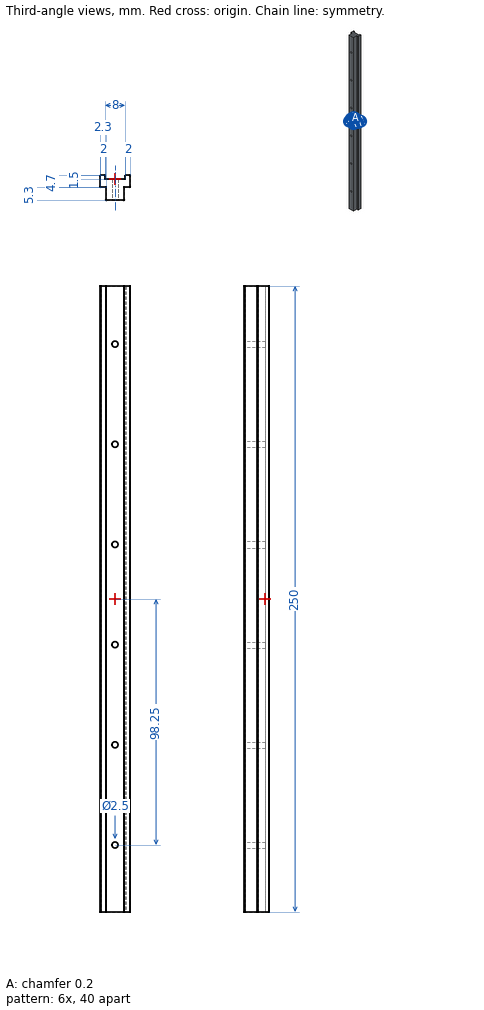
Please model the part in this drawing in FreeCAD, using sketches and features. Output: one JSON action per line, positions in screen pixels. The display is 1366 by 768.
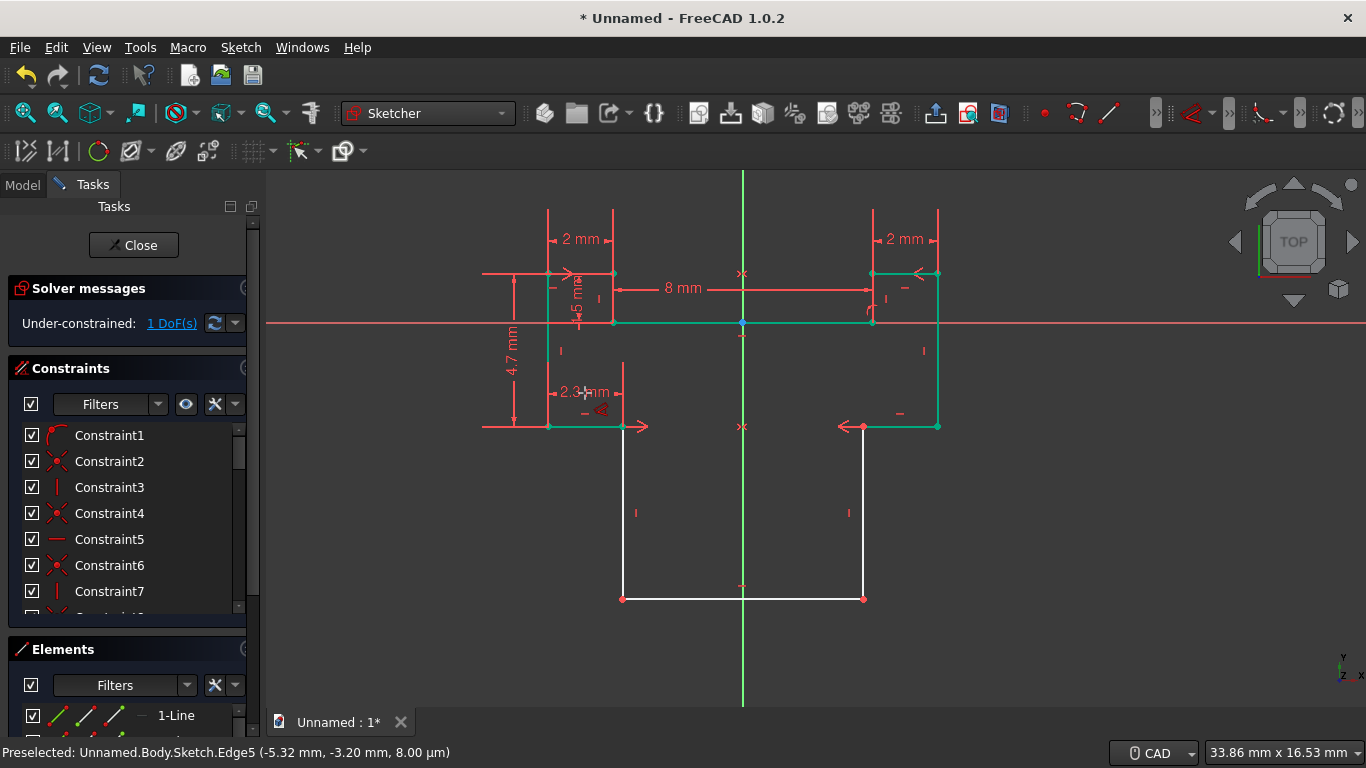
{"action": "left_click", "coordinate": [623, 478]}
{"action": "left_click", "coordinate": [589, 513]}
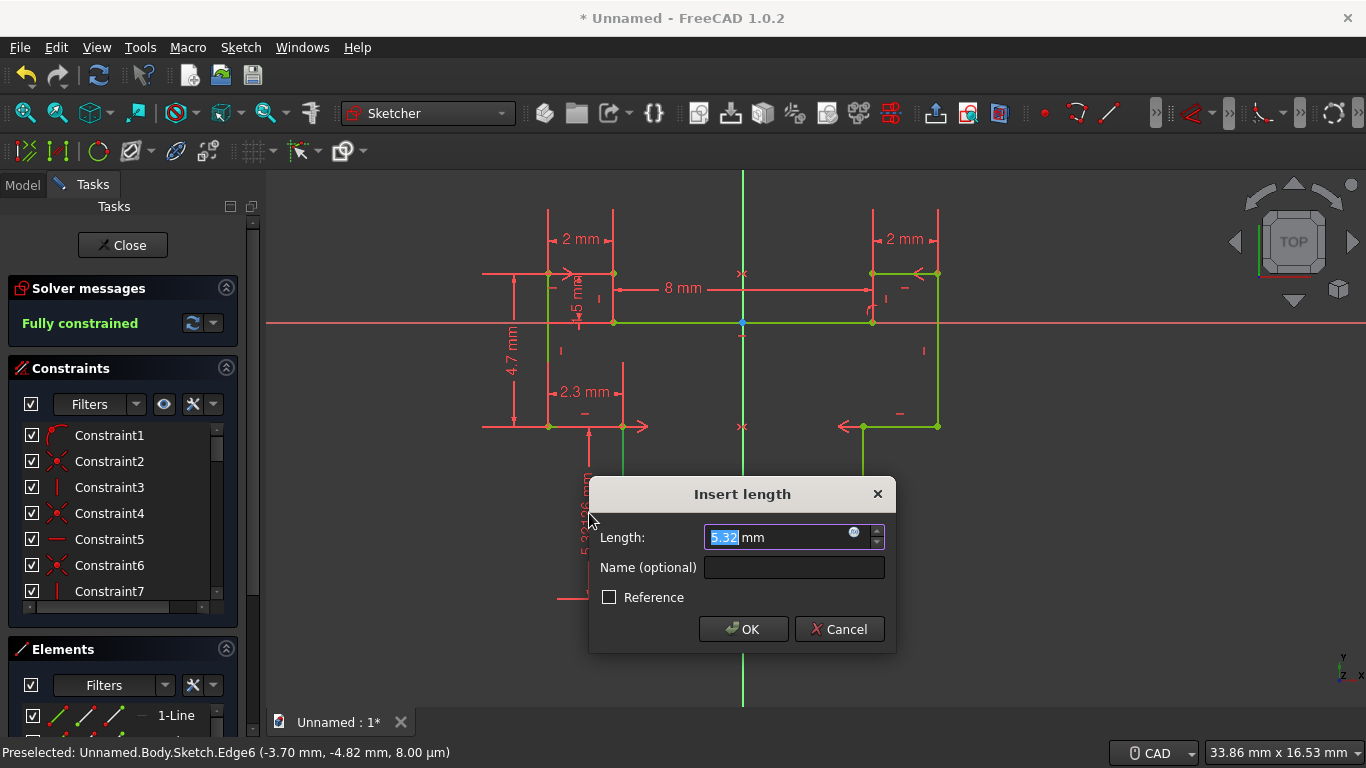
{"action": "type", "text": "5.3"}
{"action": "key", "text": "Return"}
{"action": "key", "text": "Escape"}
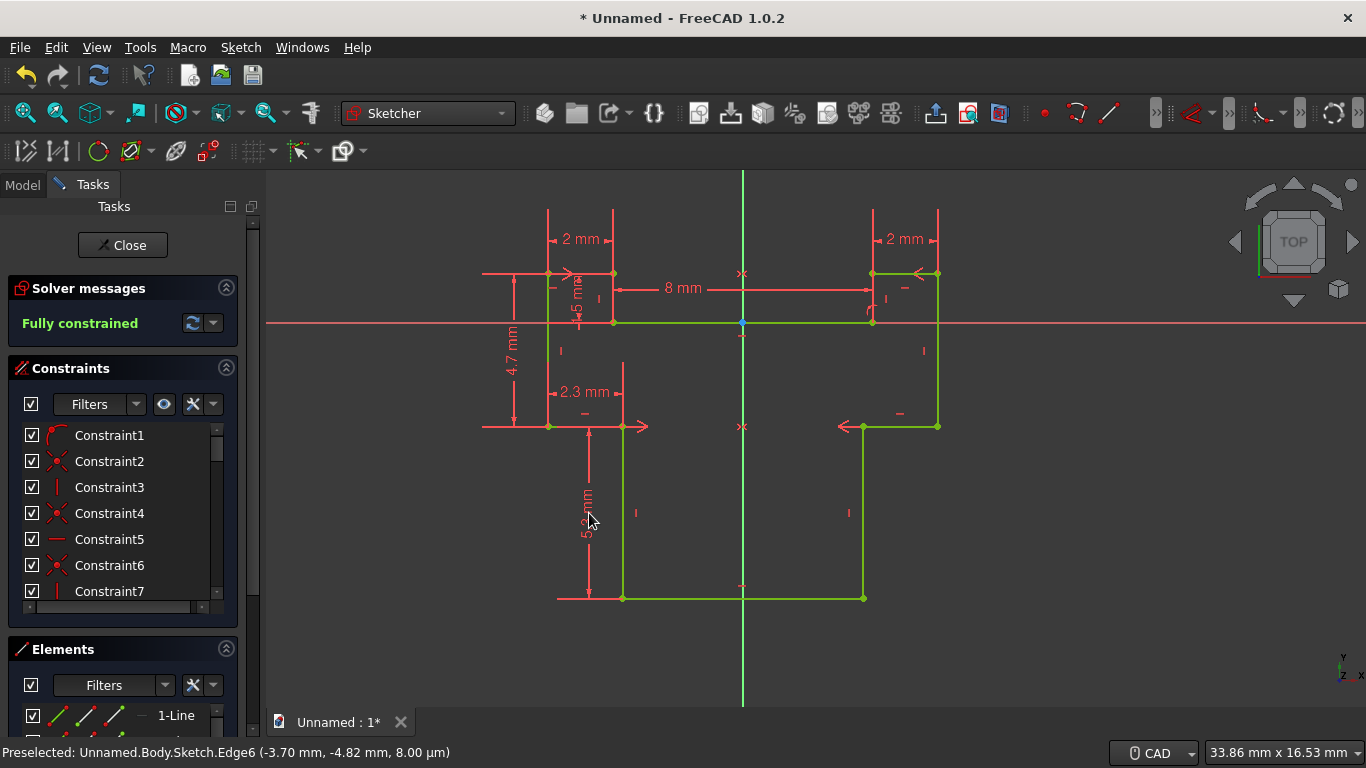
{"action": "left_click", "coordinate": [123, 245]}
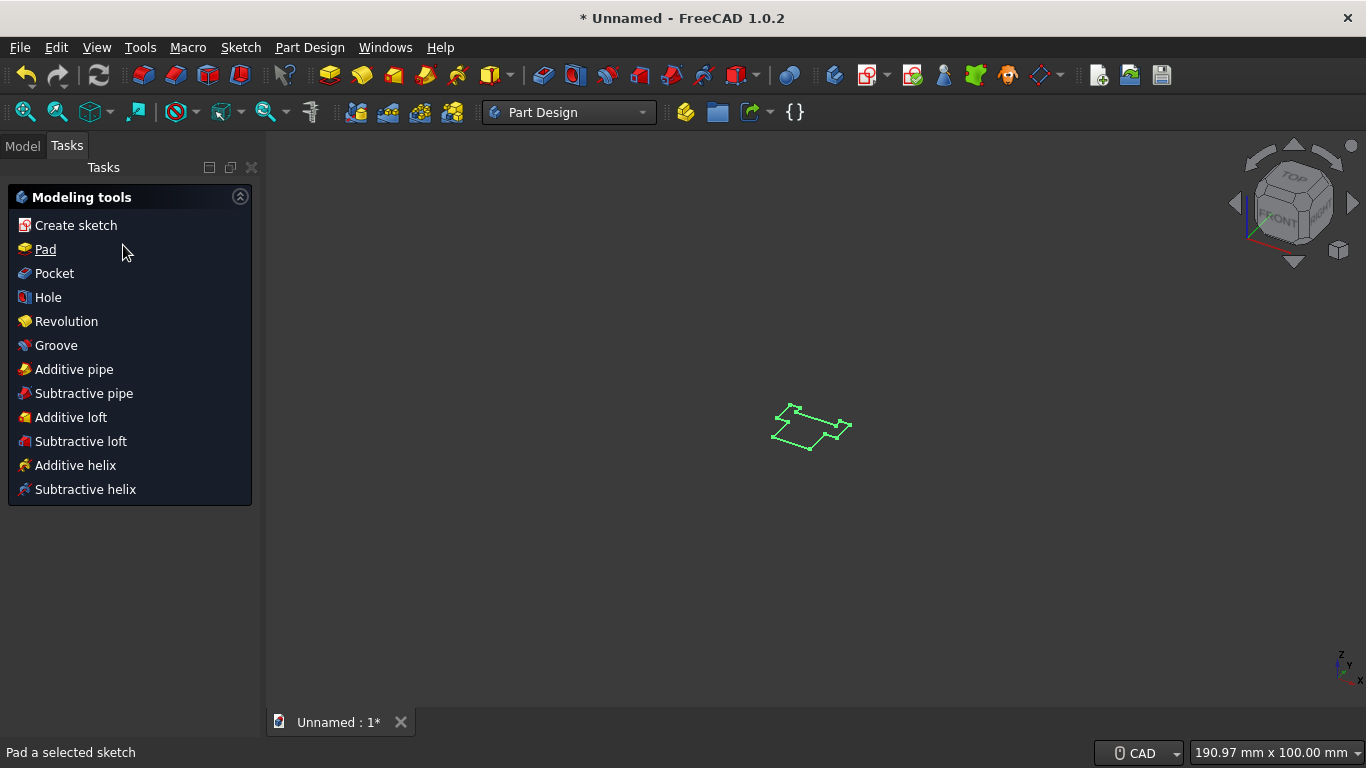
{"action": "left_click", "coordinate": [330, 76]}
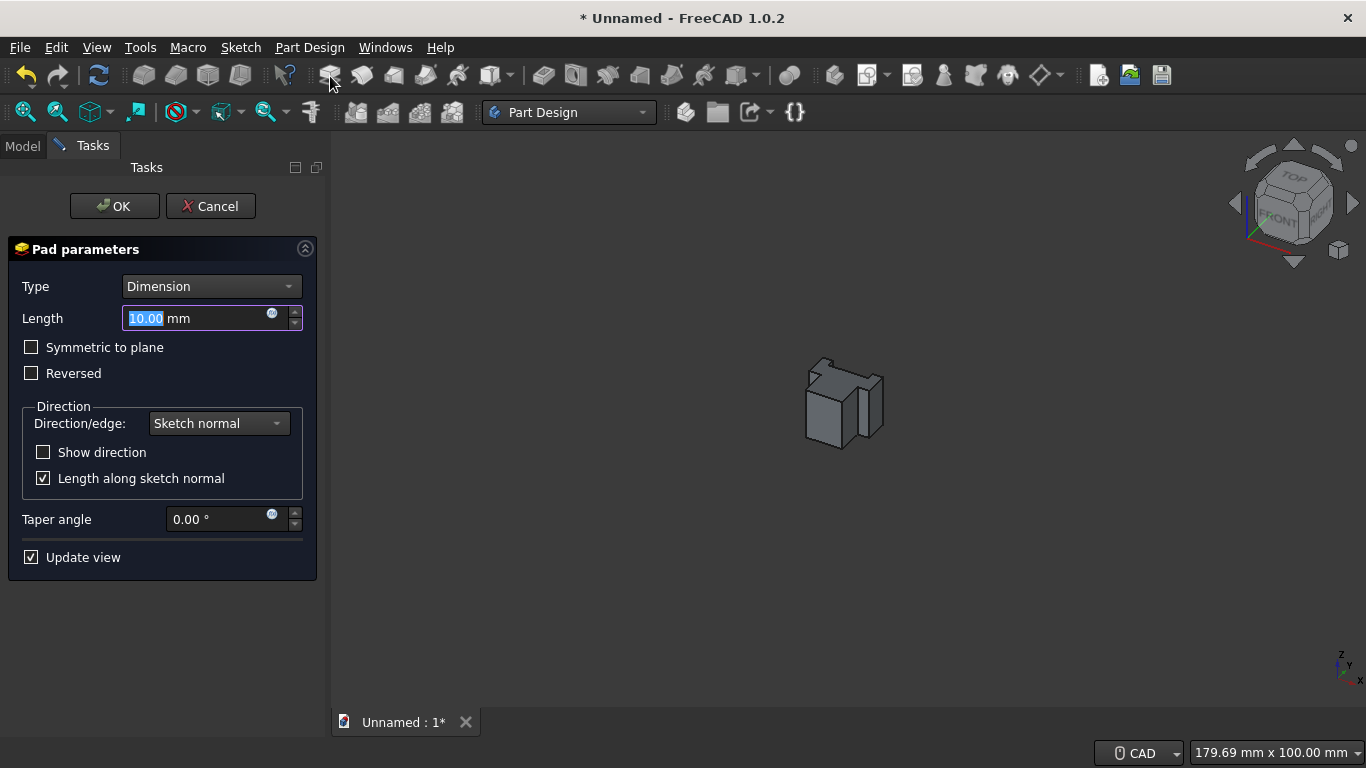
{"action": "type", "text": "250"}
{"action": "key", "text": "Tab"}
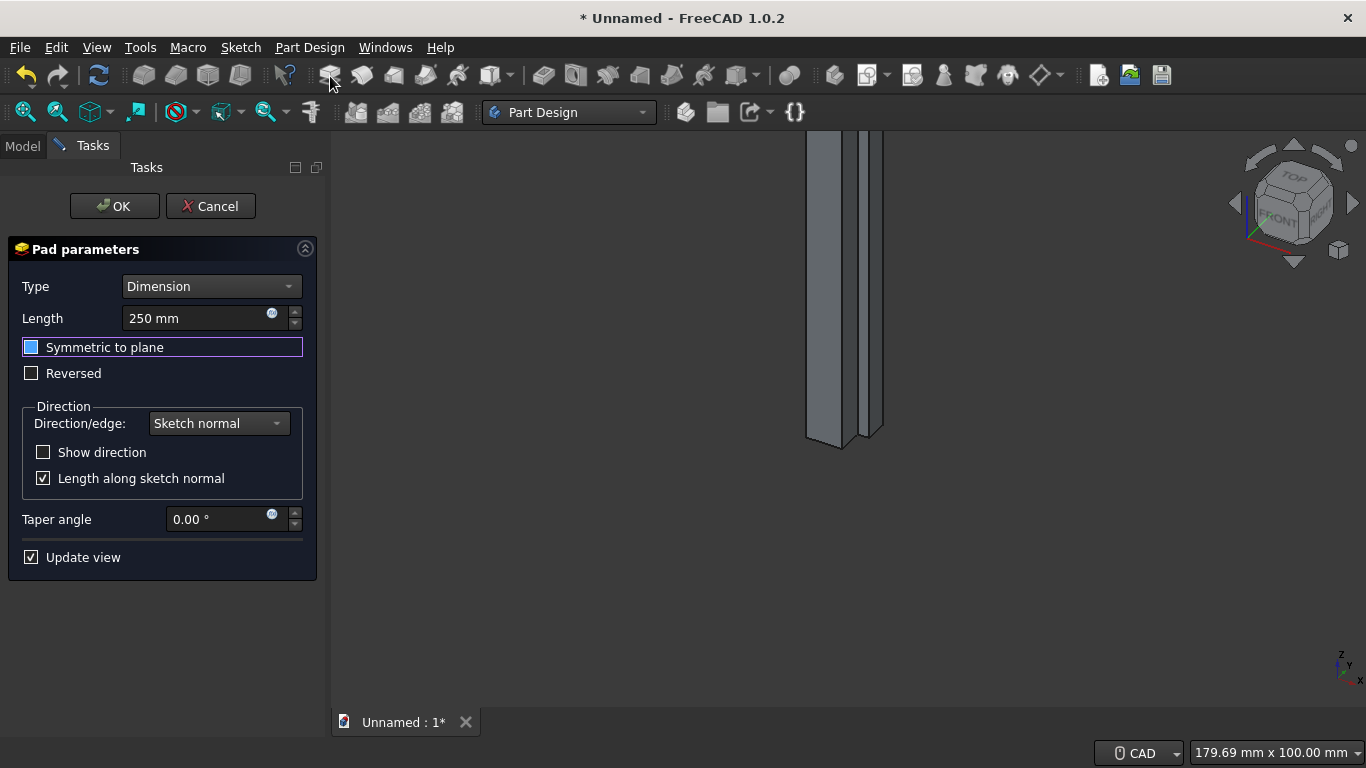
{"action": "left_click", "coordinate": [30, 347]}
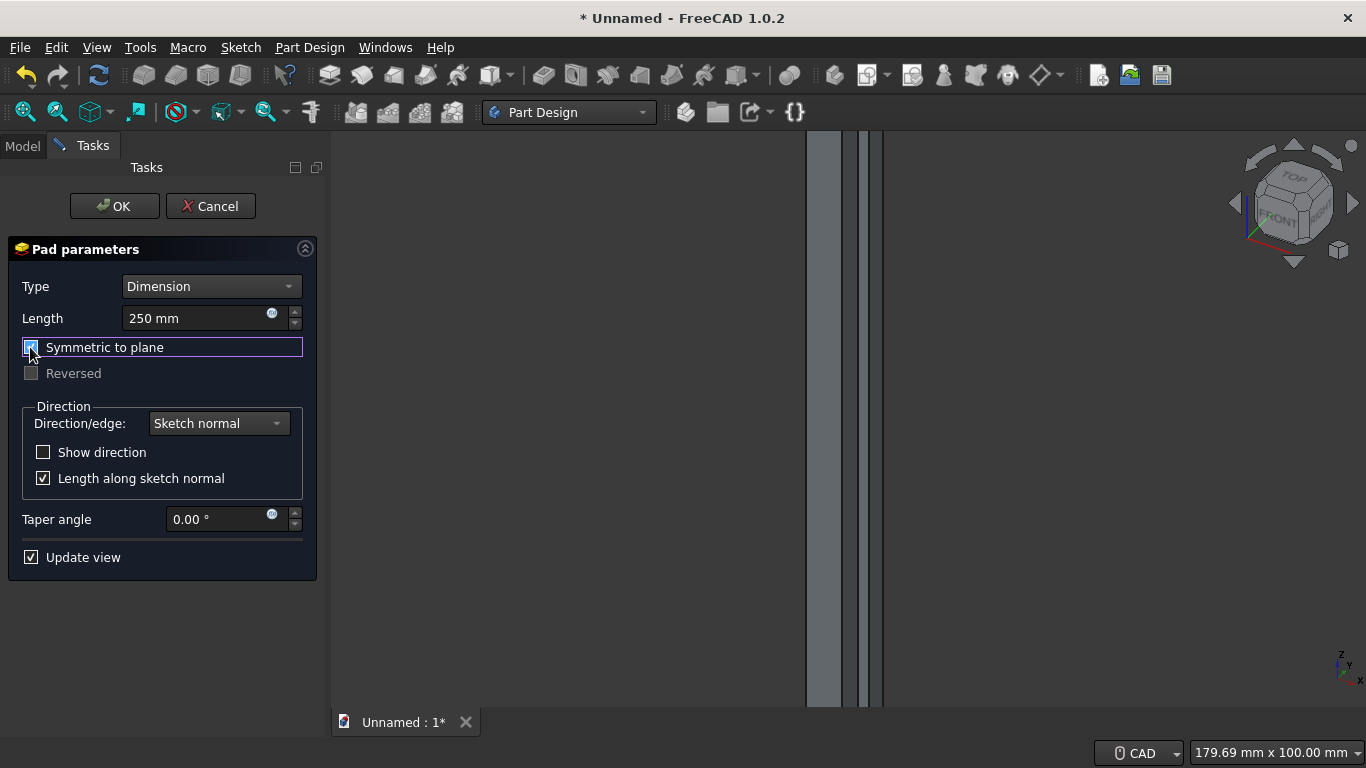
{"action": "left_click", "coordinate": [115, 206]}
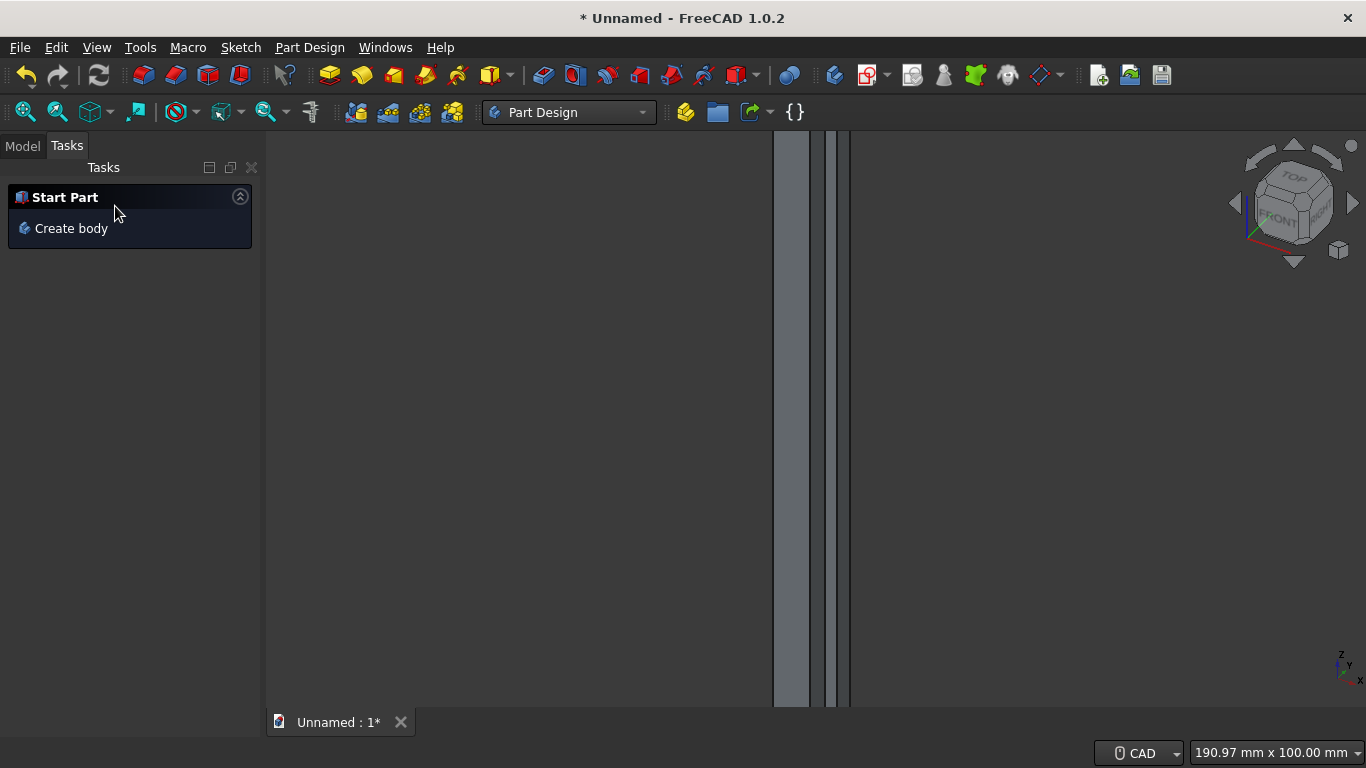
{"action": "left_click", "coordinate": [26, 112]}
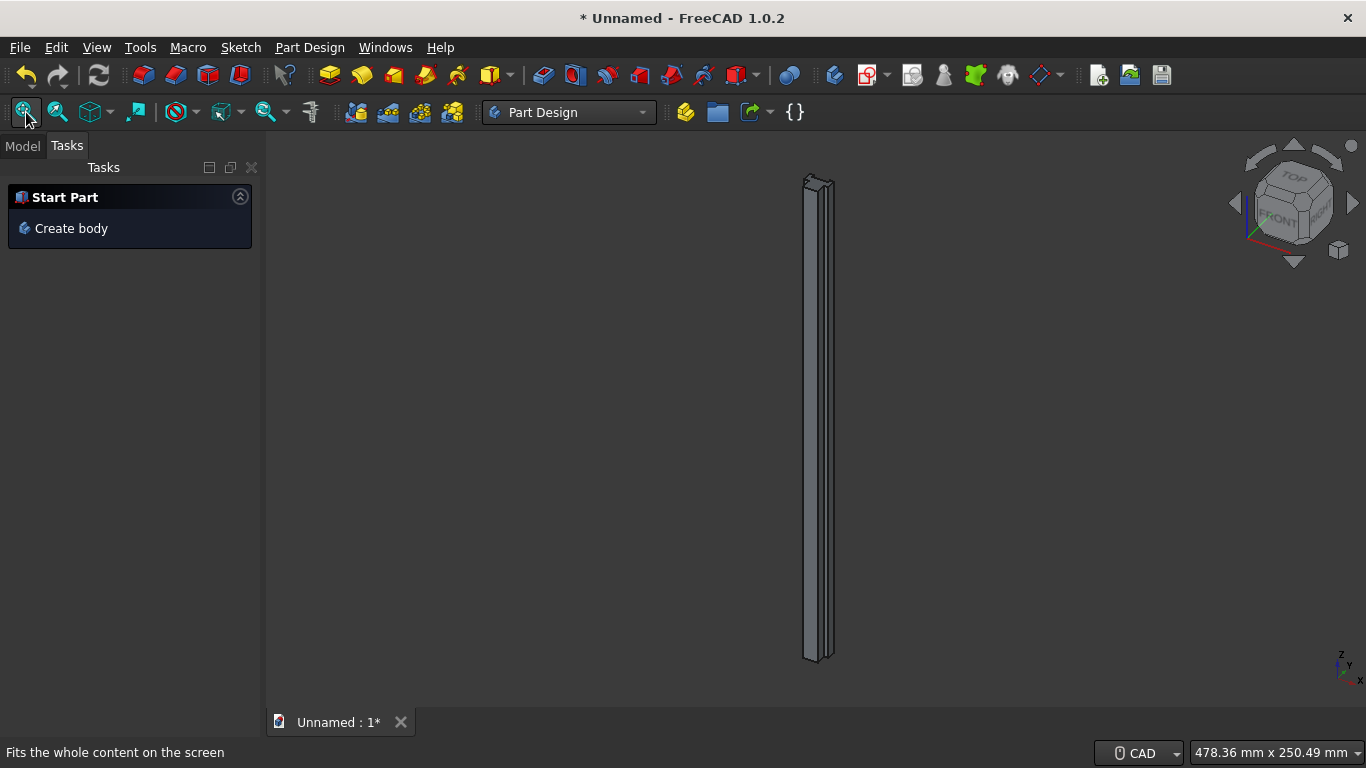
{"action": "left_click", "coordinate": [868, 76]}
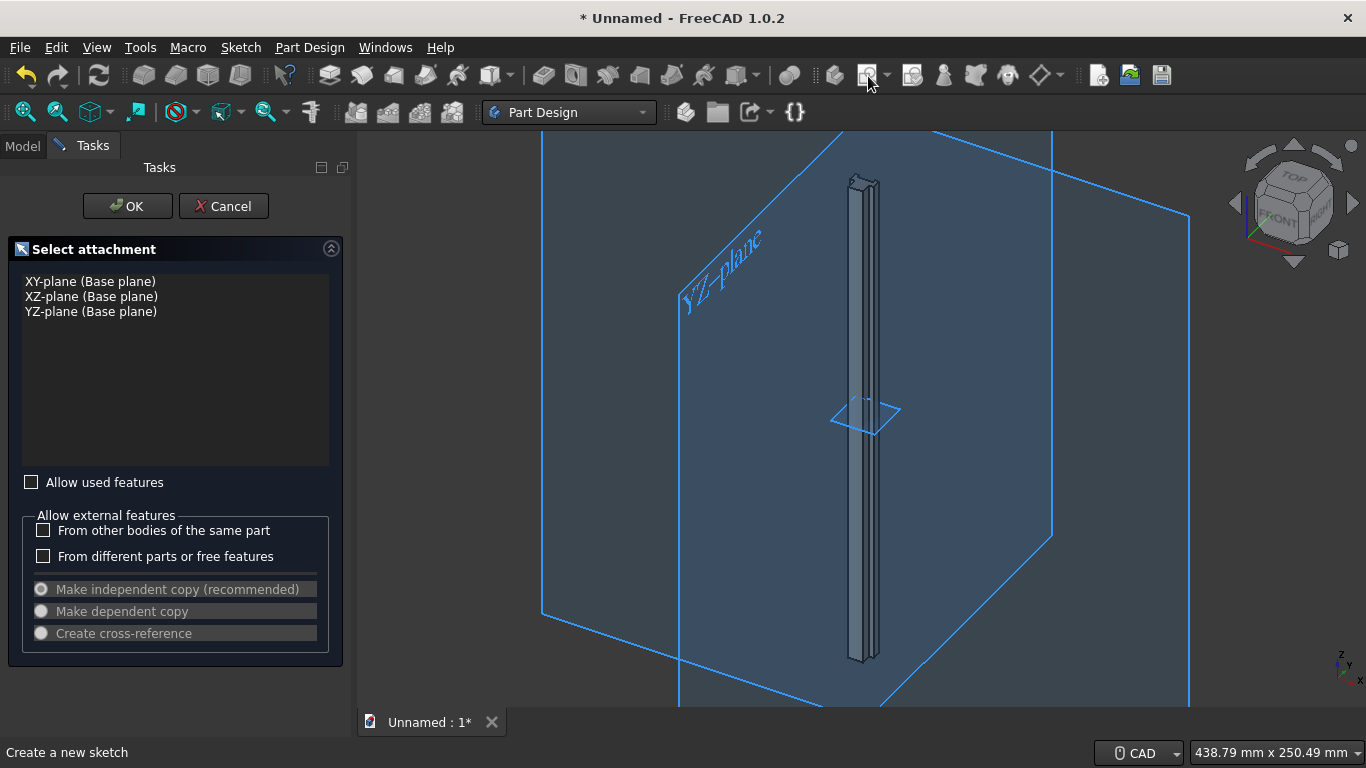
{"action": "left_click", "coordinate": [82, 296]}